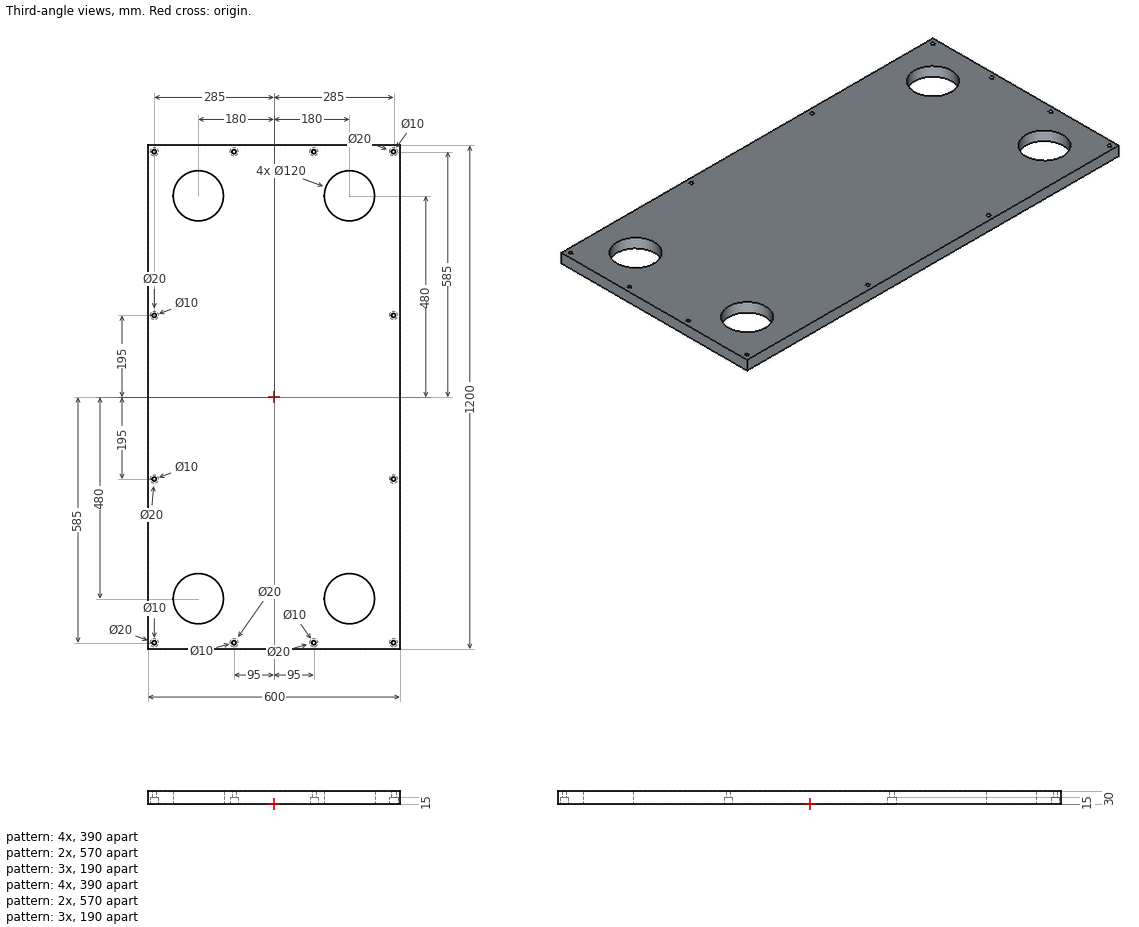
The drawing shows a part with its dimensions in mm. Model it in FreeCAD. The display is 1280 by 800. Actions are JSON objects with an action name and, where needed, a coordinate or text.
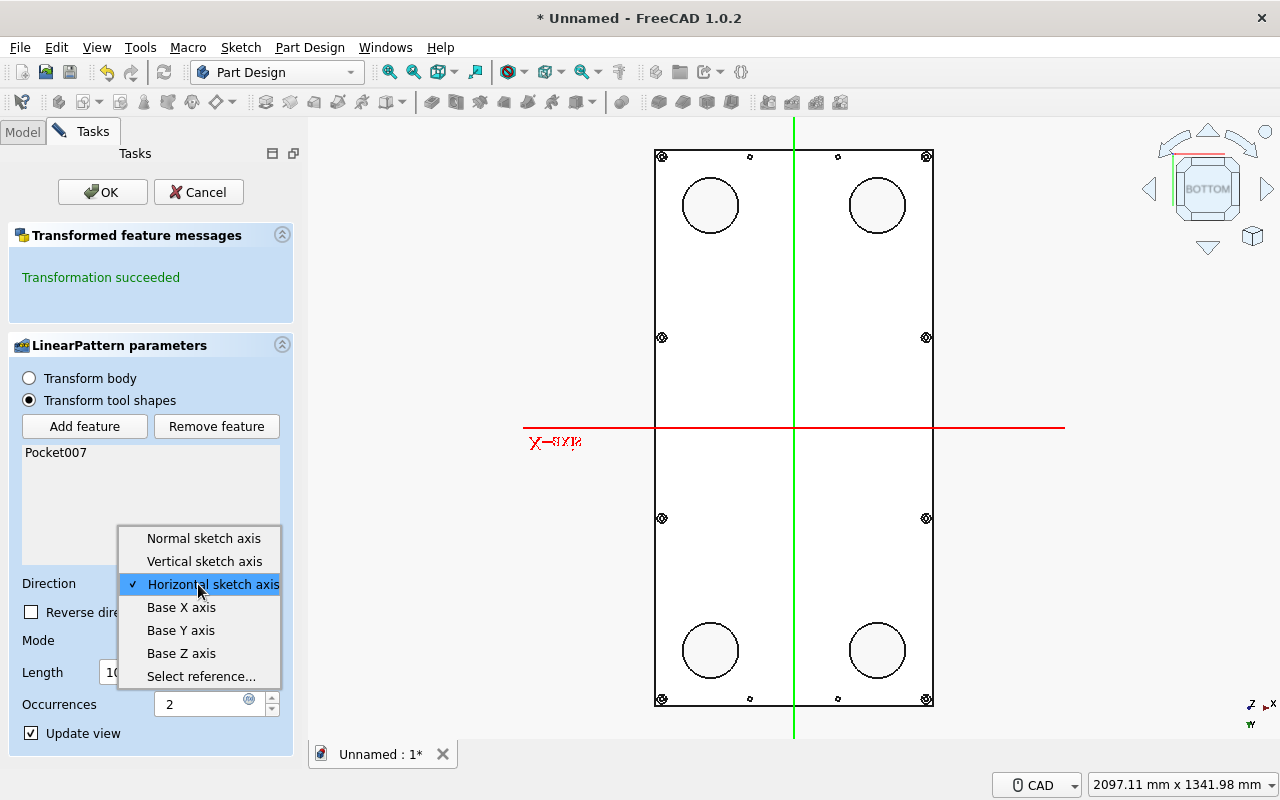
{"action": "left_click", "coordinate": [198, 608]}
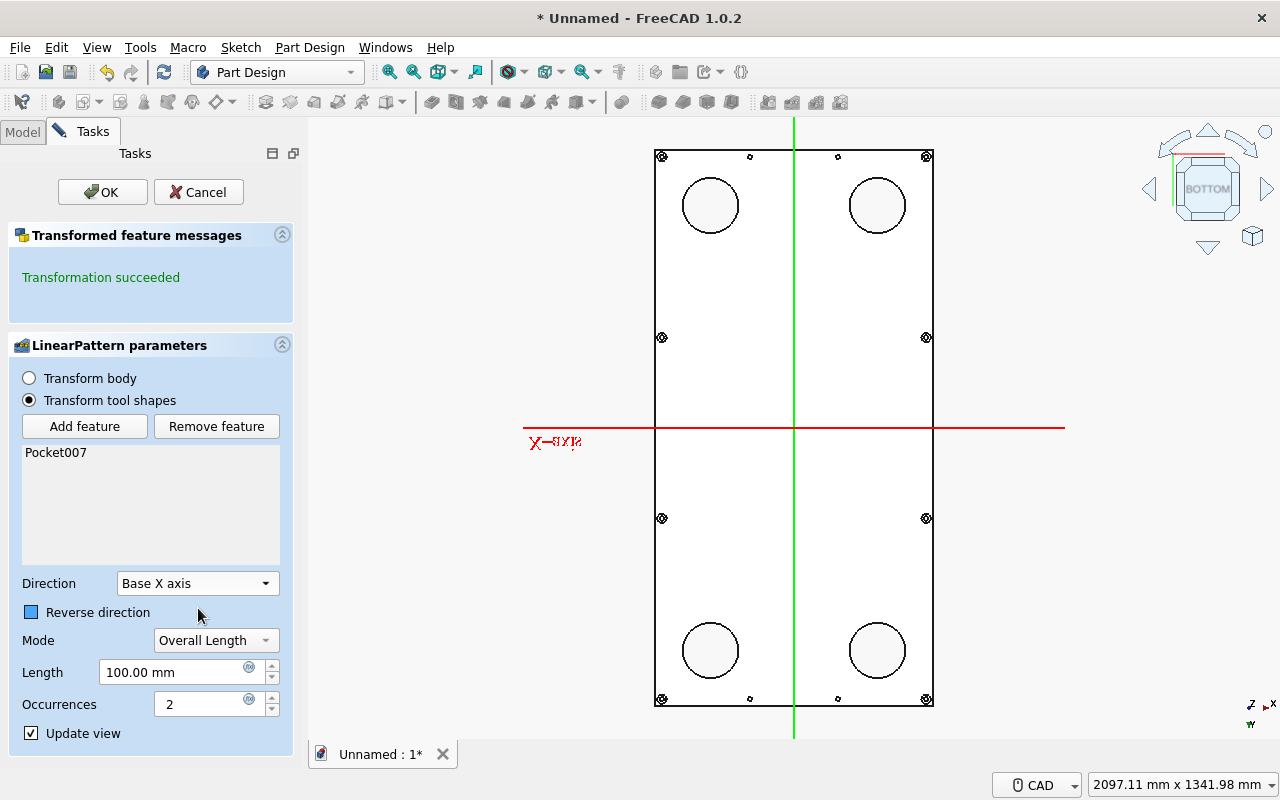
{"action": "left_click", "coordinate": [217, 640]}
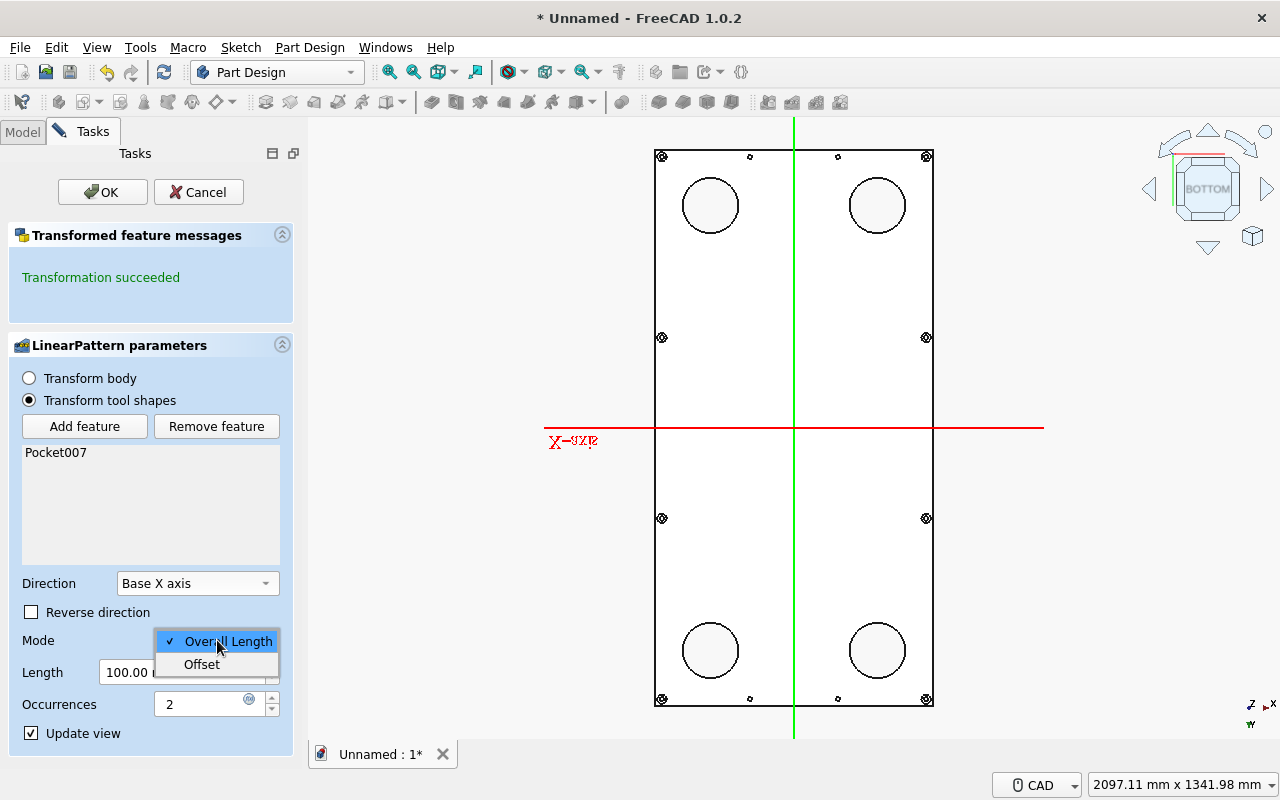
{"action": "left_click", "coordinate": [216, 664]}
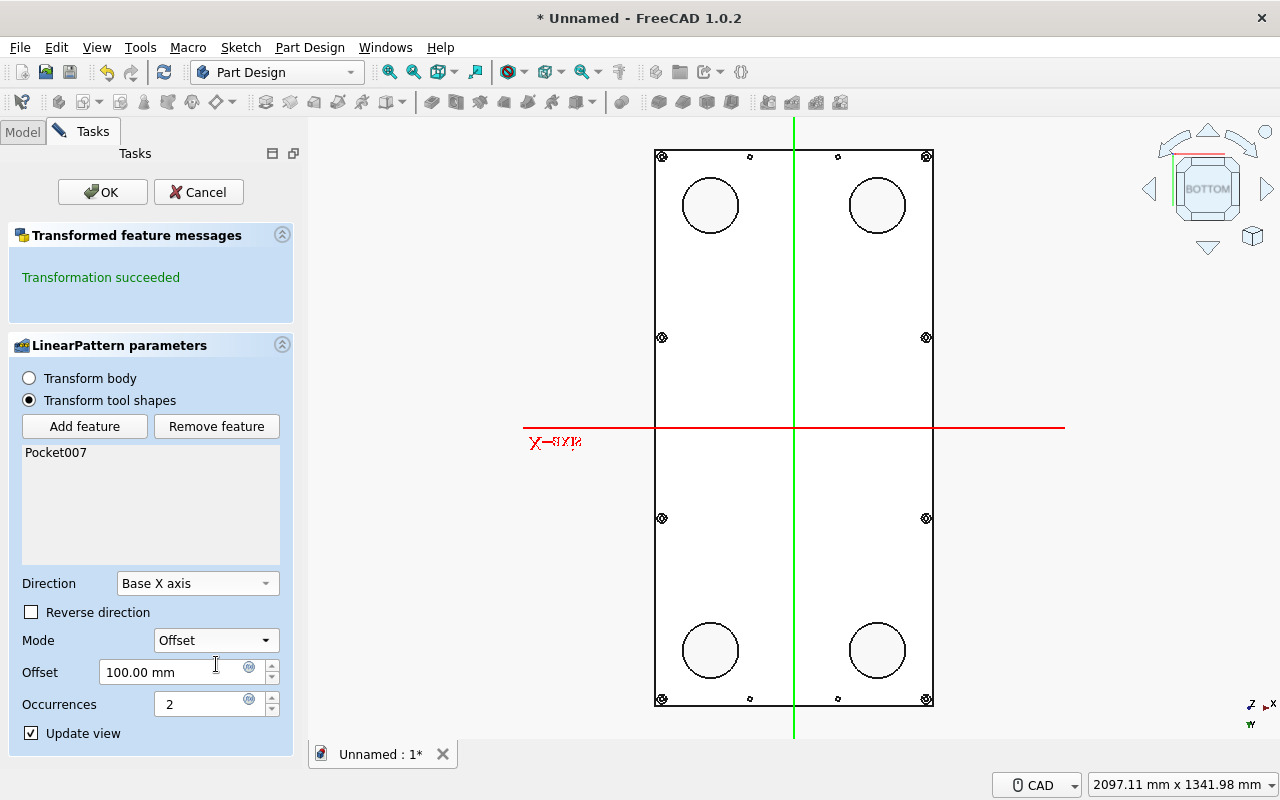
{"action": "triple_click", "coordinate": [182, 672]}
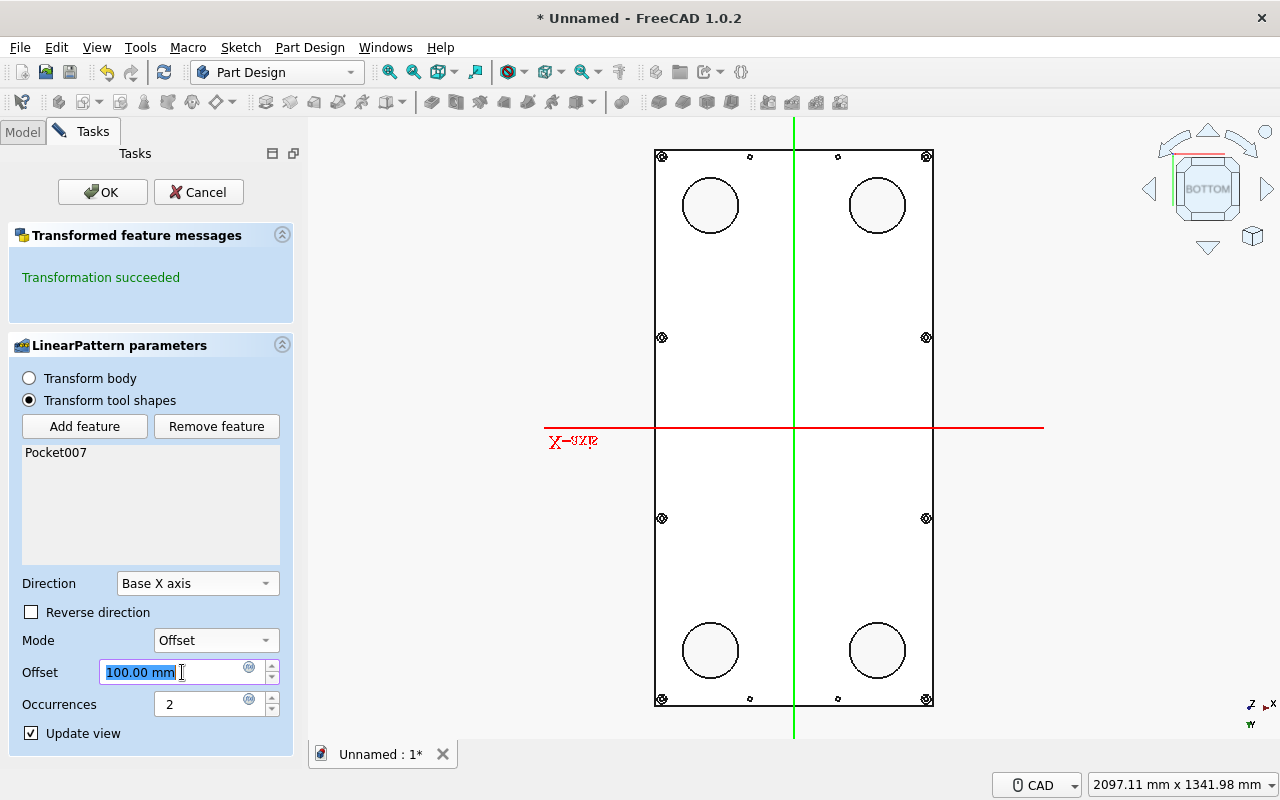
{"action": "type", "text": "190"}
{"action": "key", "text": "Tab"}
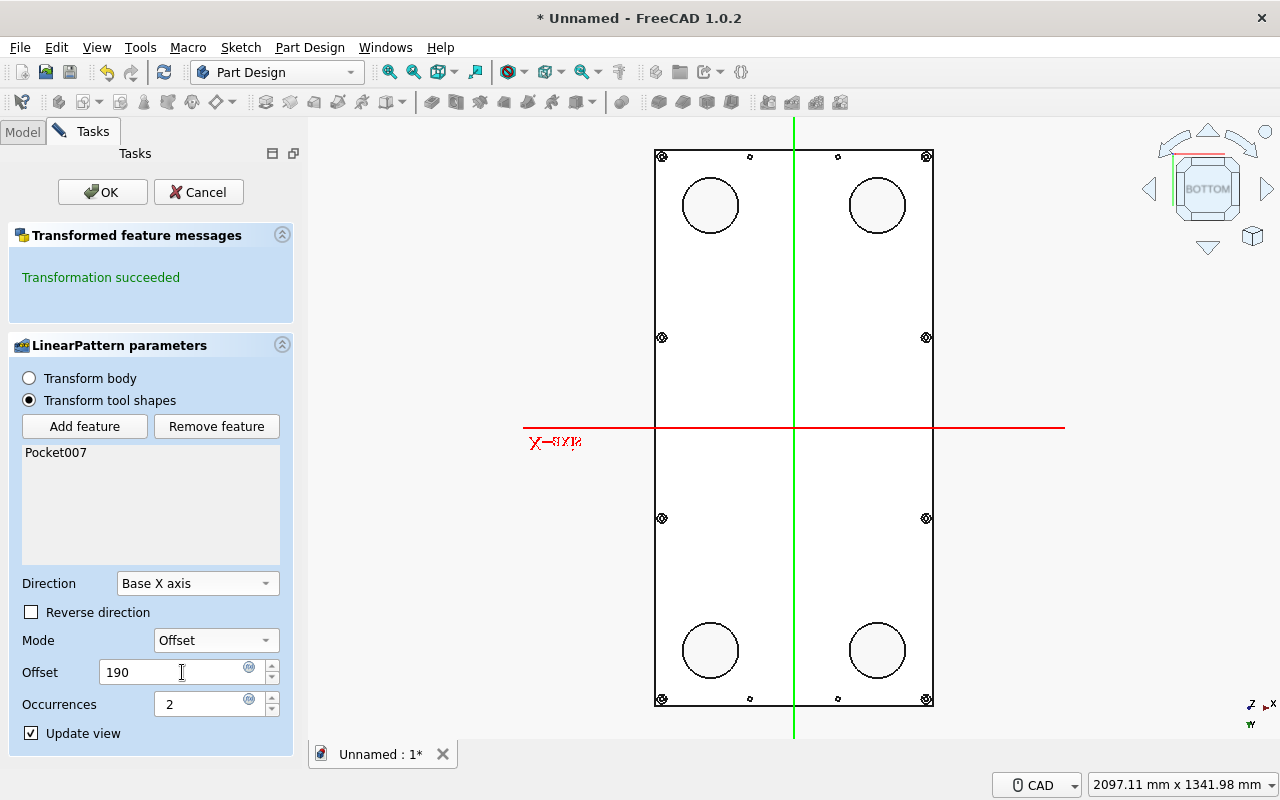
{"action": "triple_click", "coordinate": [209, 704]}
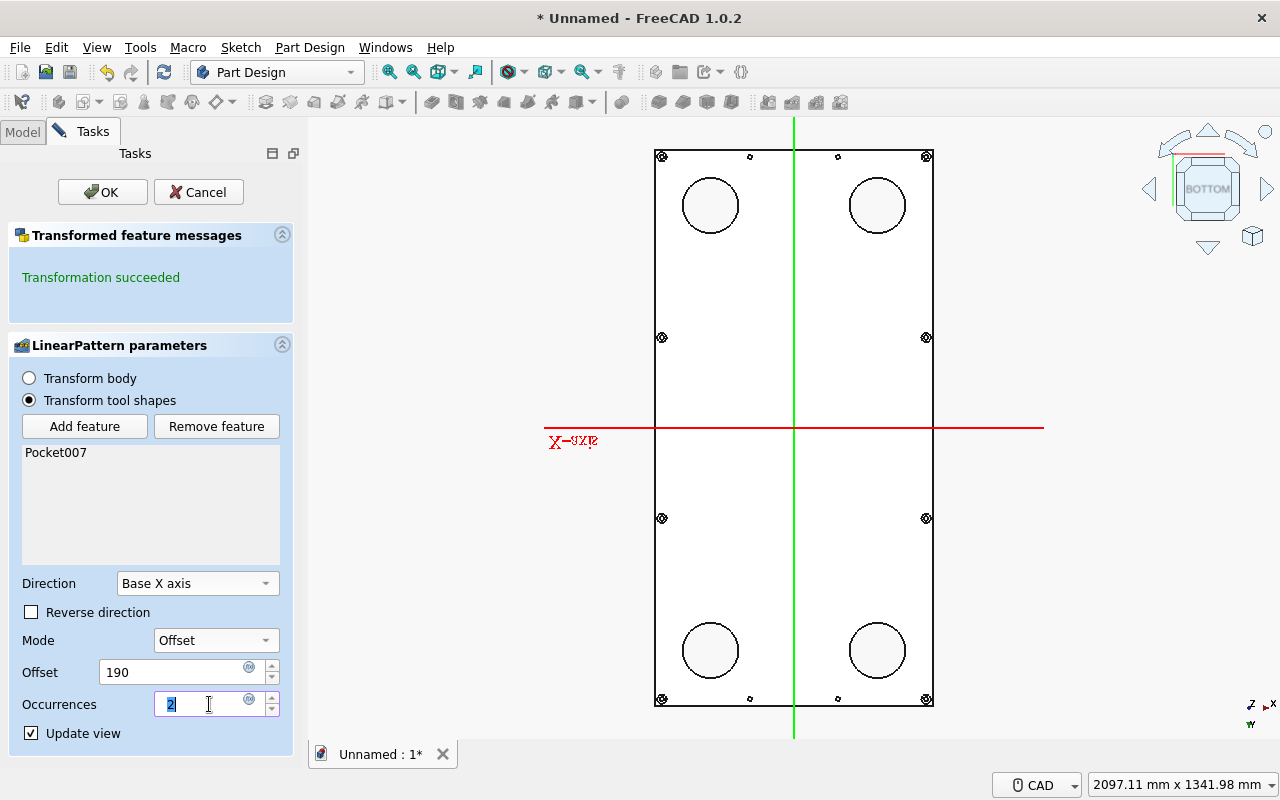
{"action": "type", "text": "3"}
{"action": "key", "text": "Tab"}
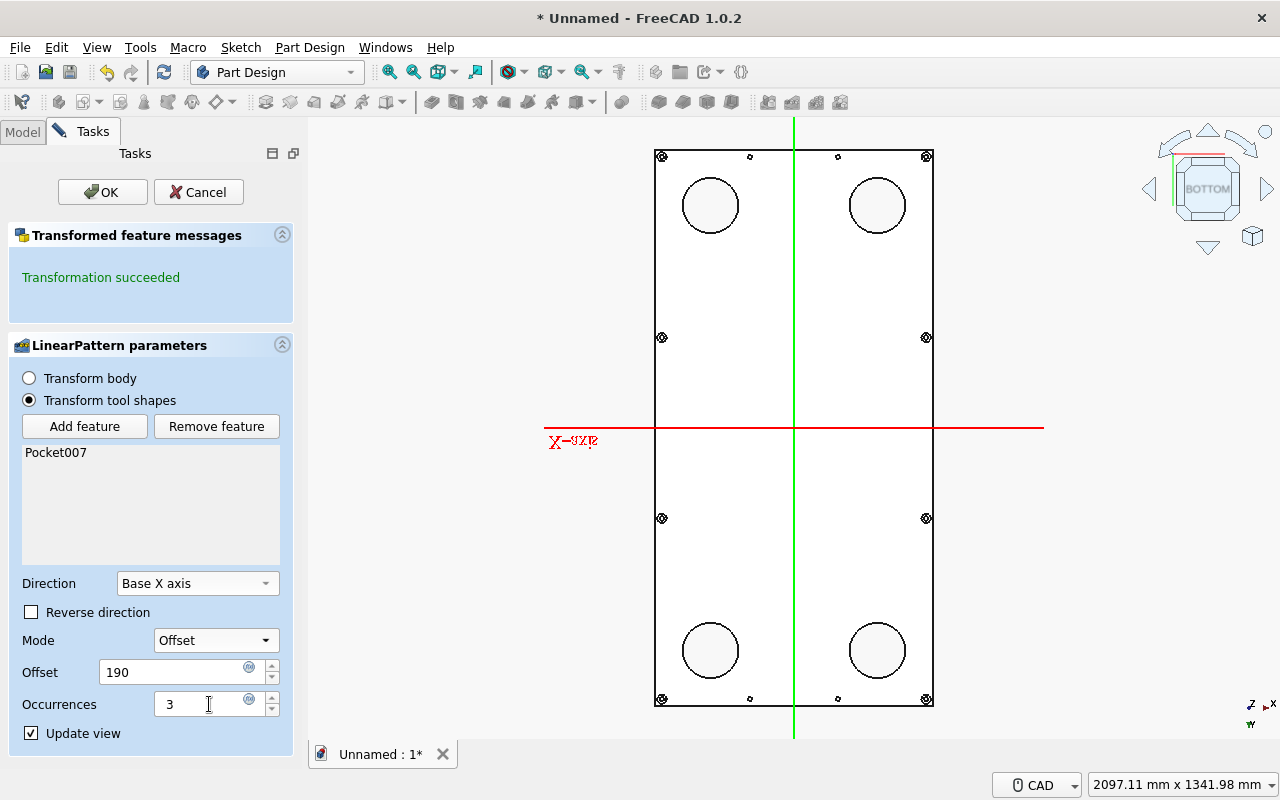
{"action": "left_click", "coordinate": [30, 612]}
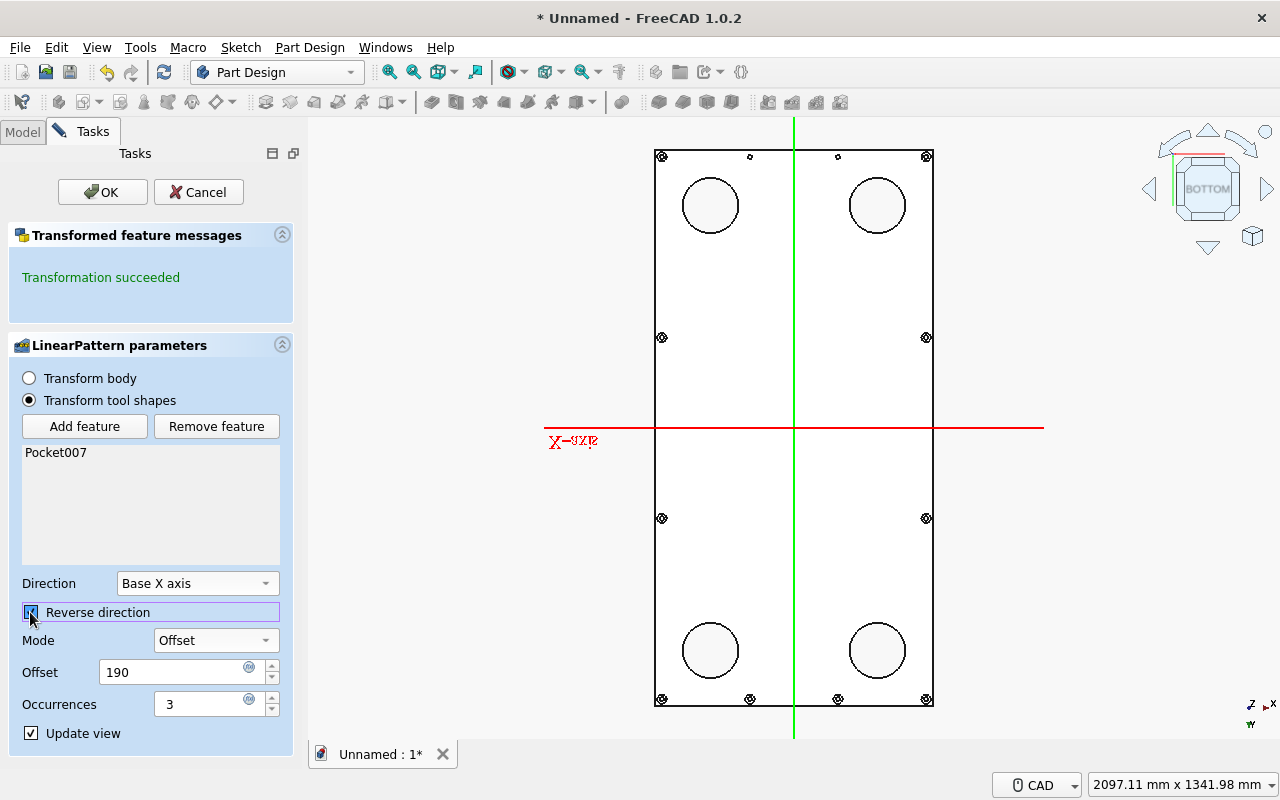
{"action": "left_click", "coordinate": [103, 192]}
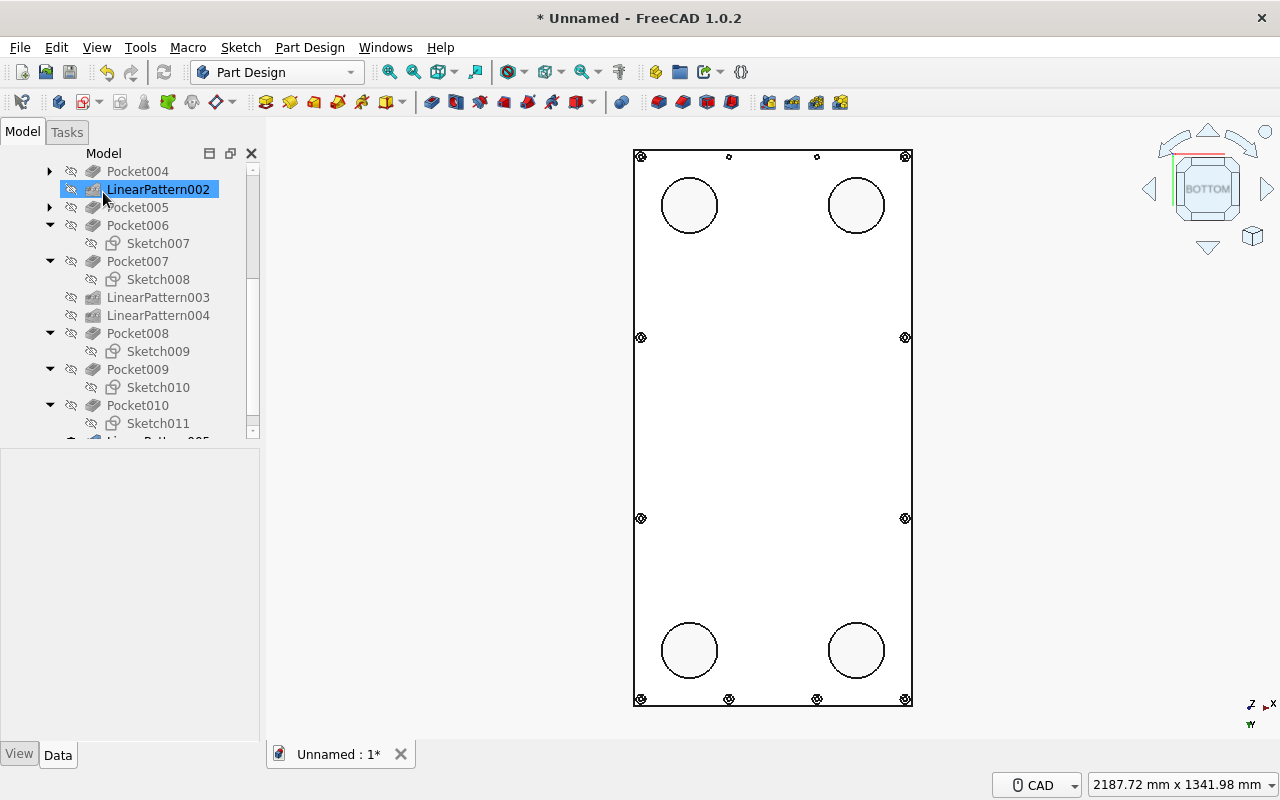
{"action": "left_click", "coordinate": [84, 102]}